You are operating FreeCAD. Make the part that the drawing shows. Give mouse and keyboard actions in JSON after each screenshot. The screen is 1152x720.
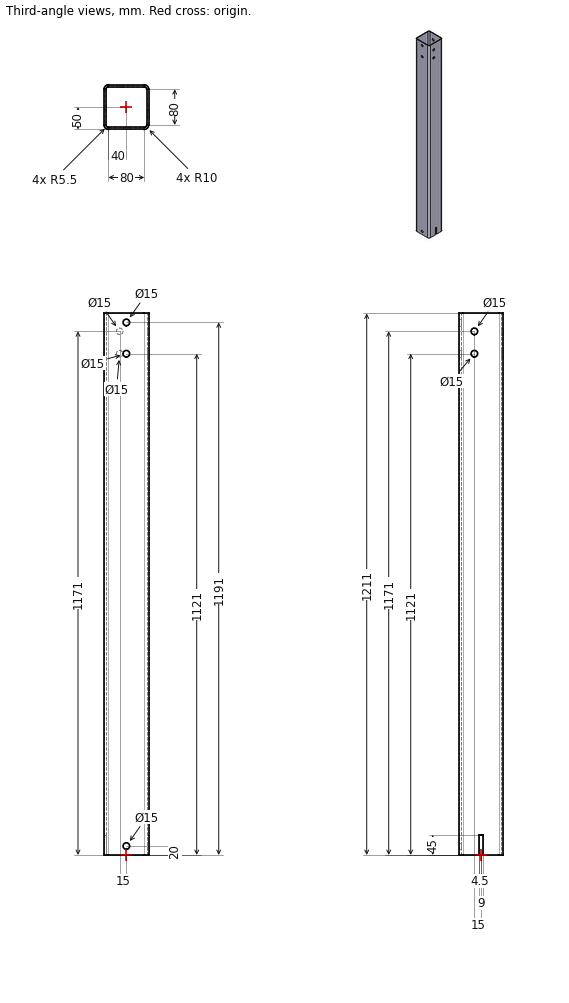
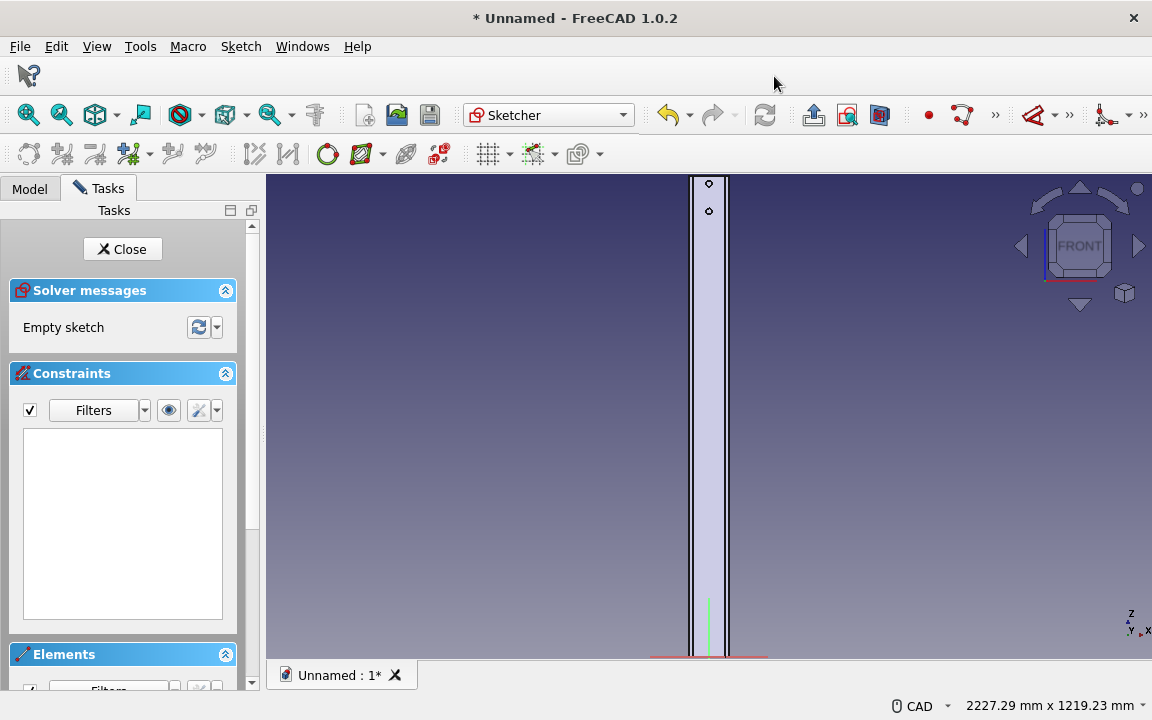
{"action": "scroll", "coordinate": [640, 416], "scroll_direction": "down", "scroll_amount": 5}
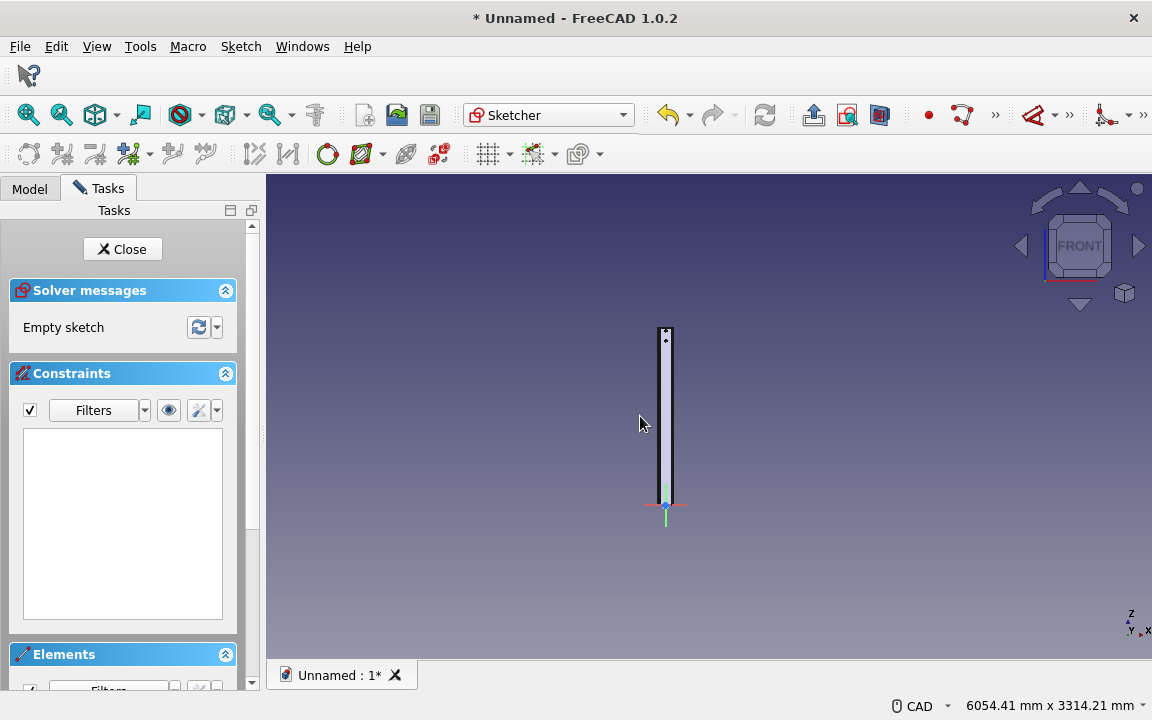
{"action": "scroll", "coordinate": [667, 508], "scroll_direction": "up", "scroll_amount": 15}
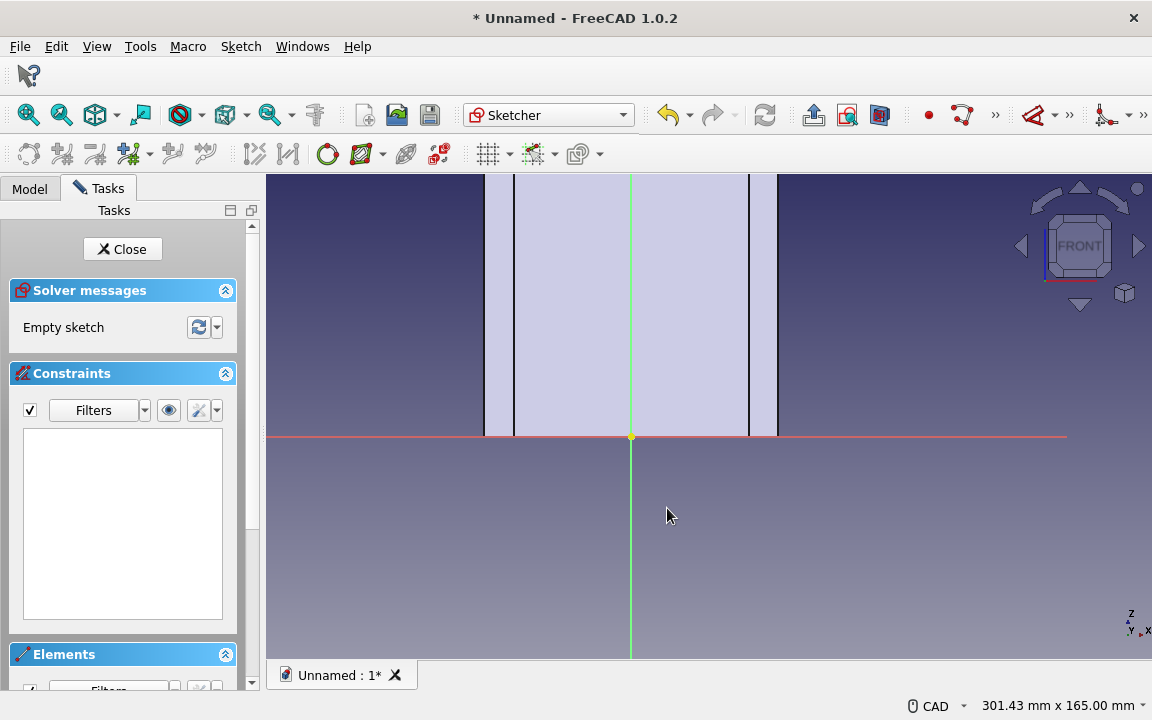
{"action": "scroll", "coordinate": [628, 390], "scroll_direction": "up", "scroll_amount": 7}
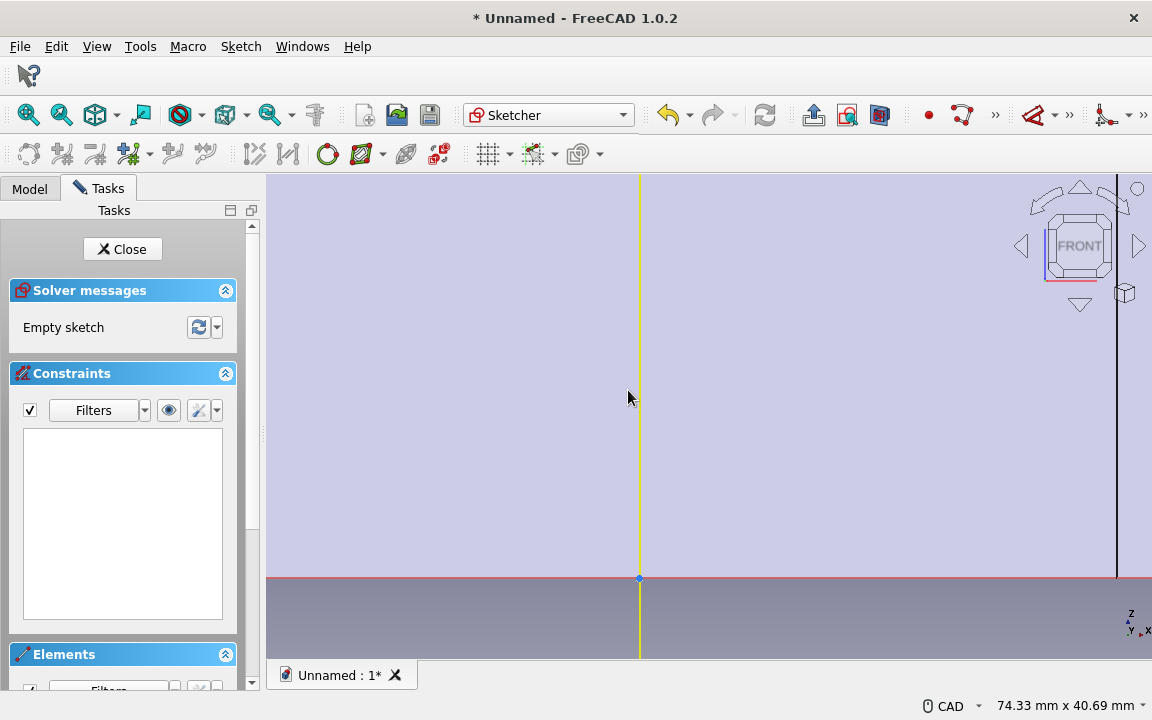
{"action": "key", "text": "g c"}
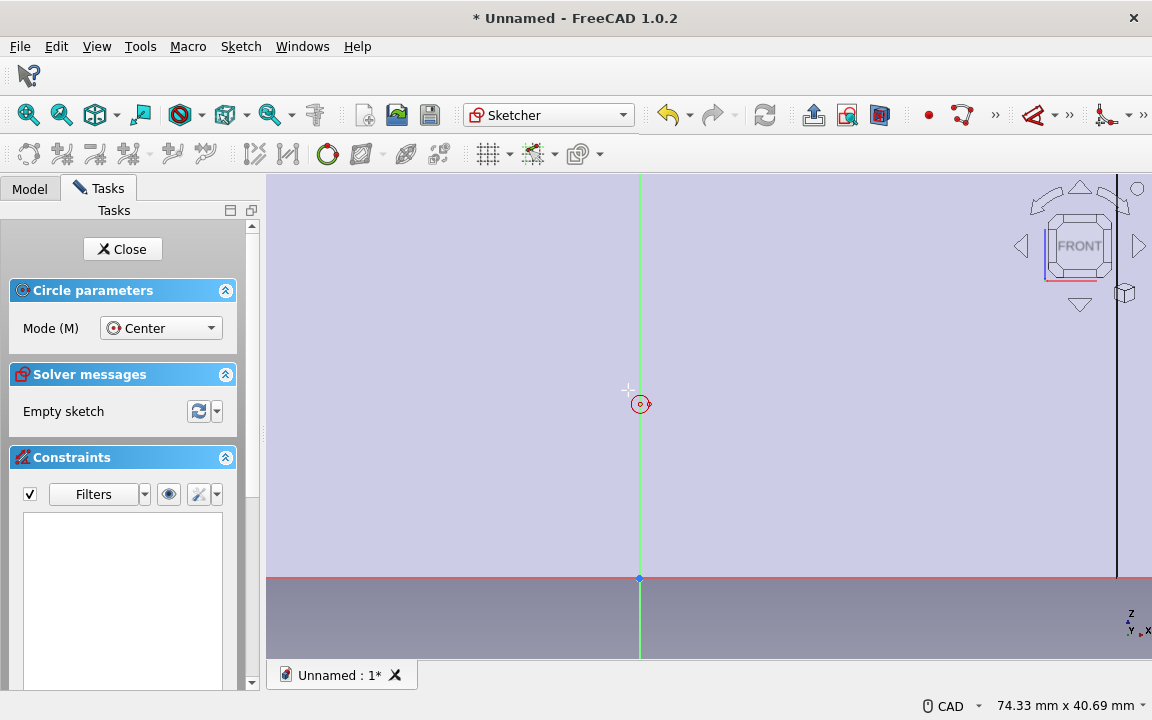
{"action": "left_click", "coordinate": [640, 340]}
{"action": "left_click", "coordinate": [703, 277]}
{"action": "key", "text": "Escape"}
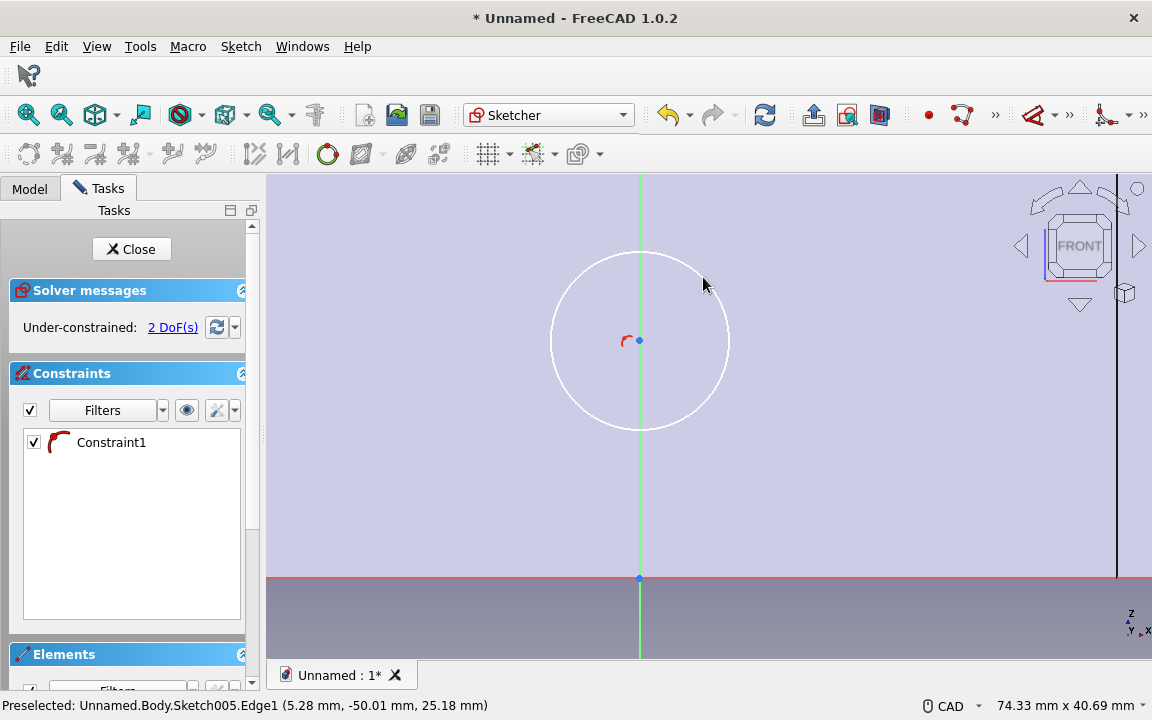
{"action": "key", "text": "d"}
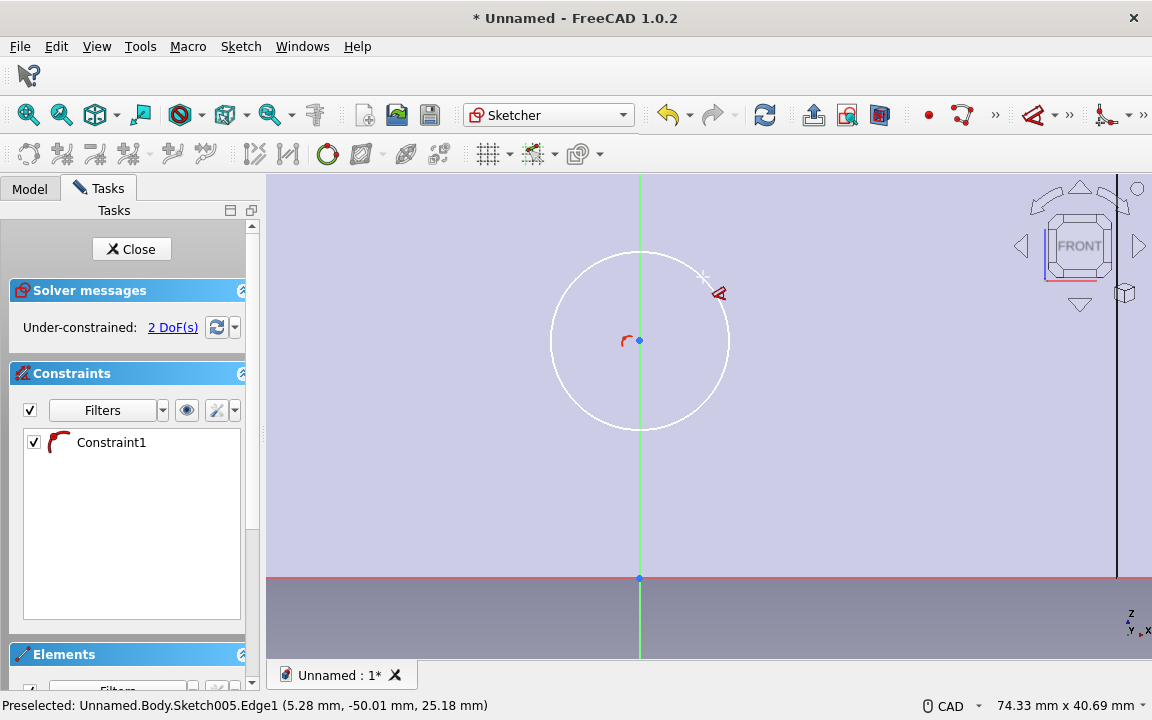
{"action": "left_click", "coordinate": [703, 278]}
{"action": "left_click", "coordinate": [726, 255]}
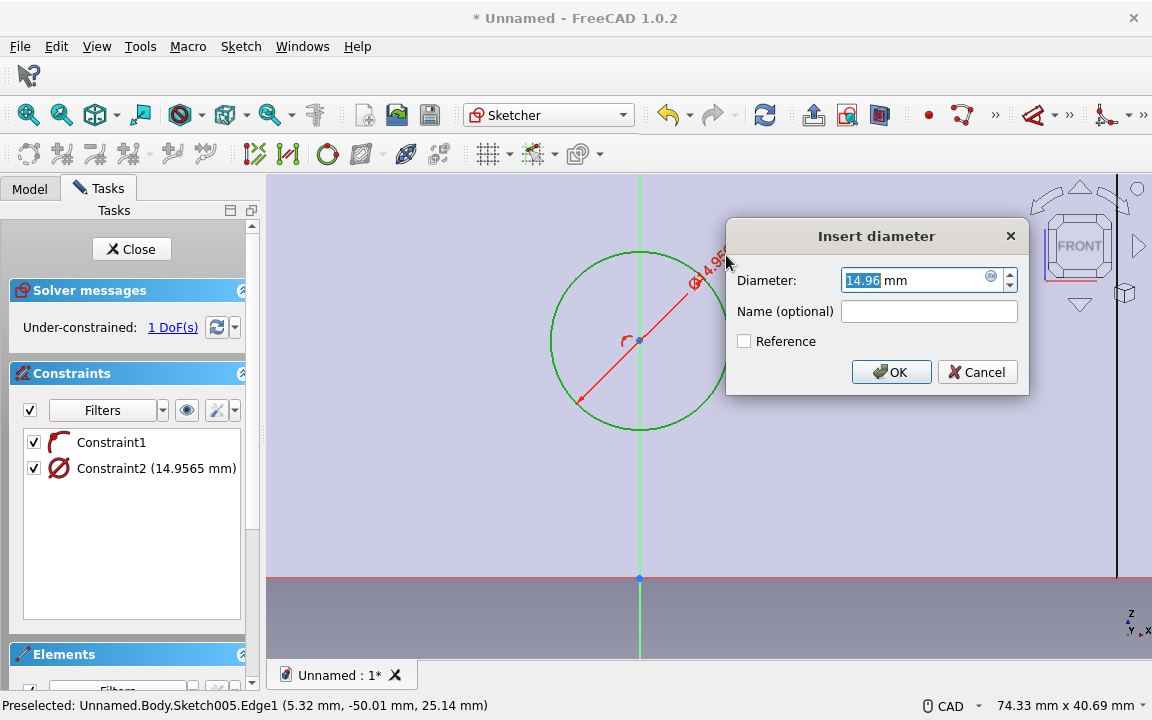
{"action": "type", "text": "15"}
{"action": "key", "text": "Return"}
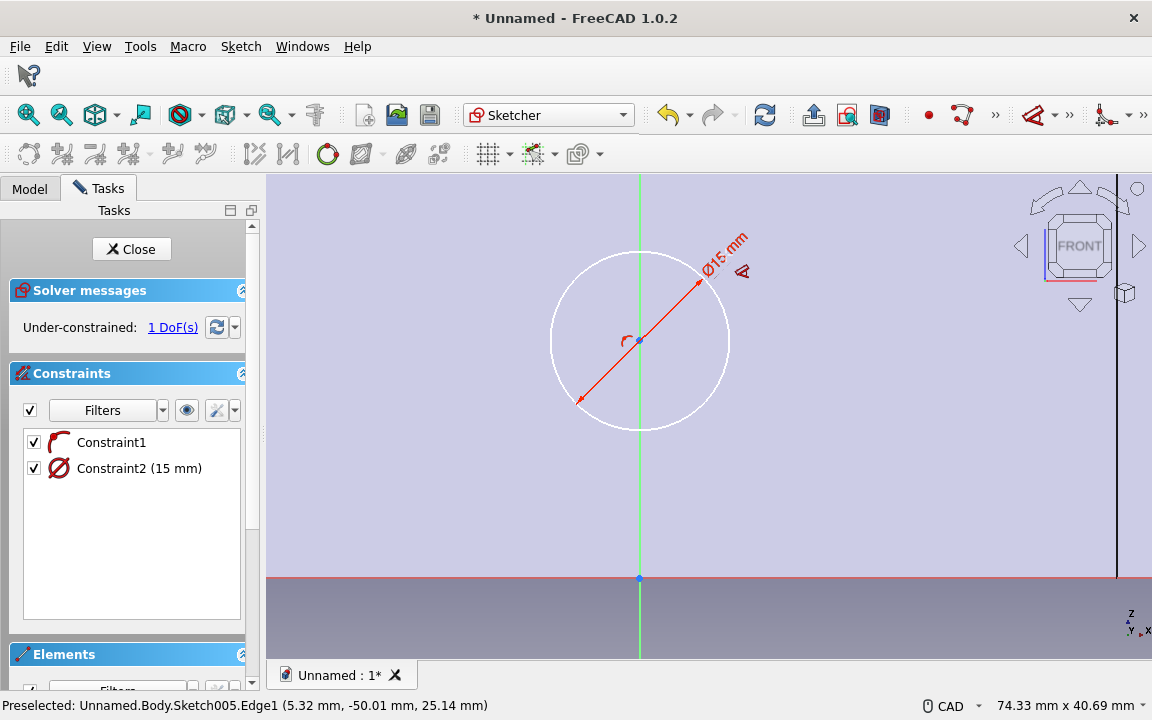
{"action": "left_click", "coordinate": [640, 341]}
{"action": "left_click", "coordinate": [674, 460]}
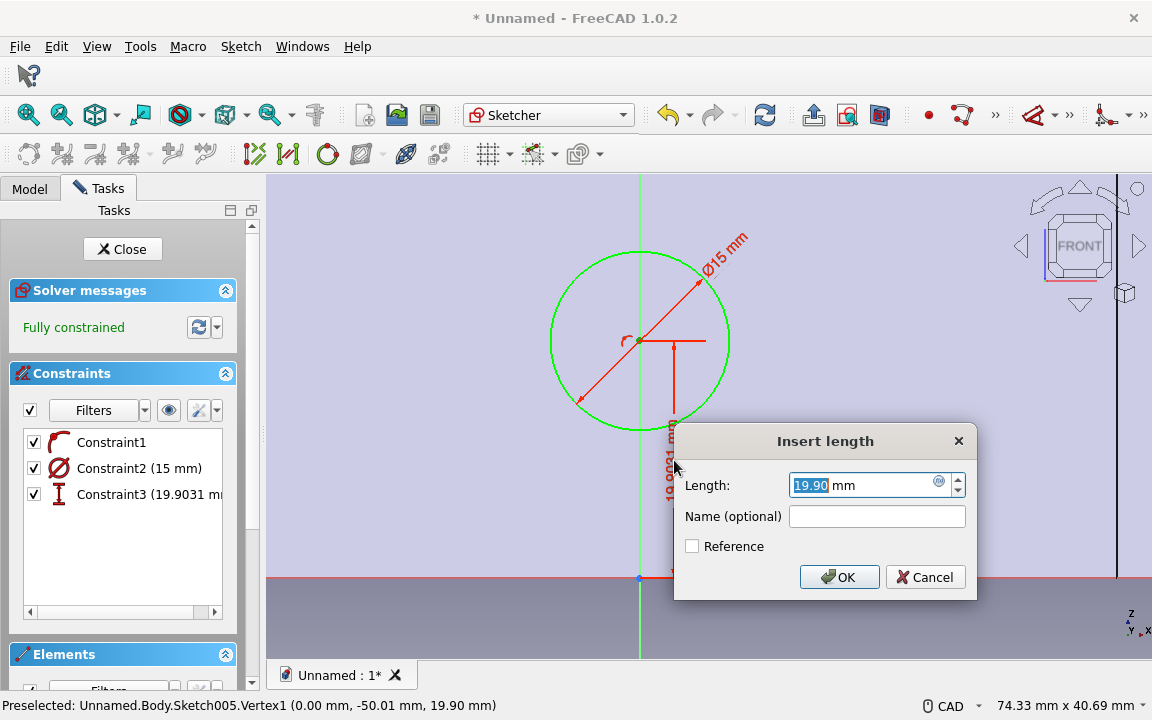
{"action": "type", "text": "20"}
{"action": "key", "text": "Return"}
{"action": "key", "text": "Escape"}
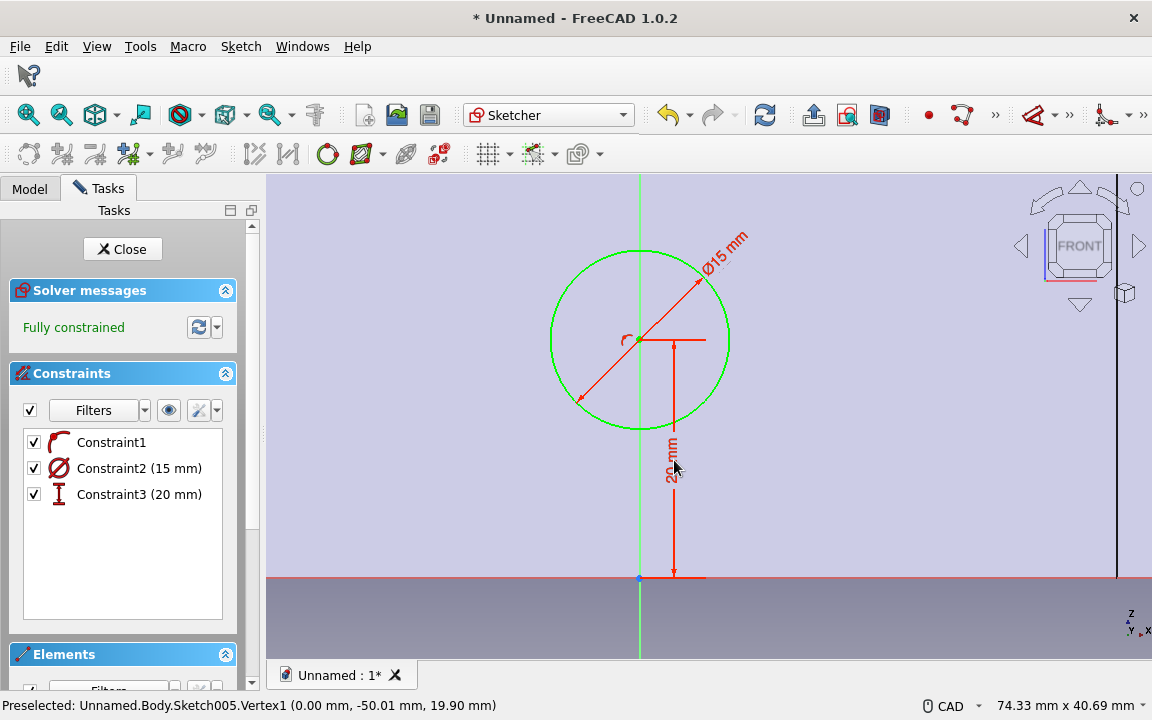
{"action": "left_click", "coordinate": [123, 249]}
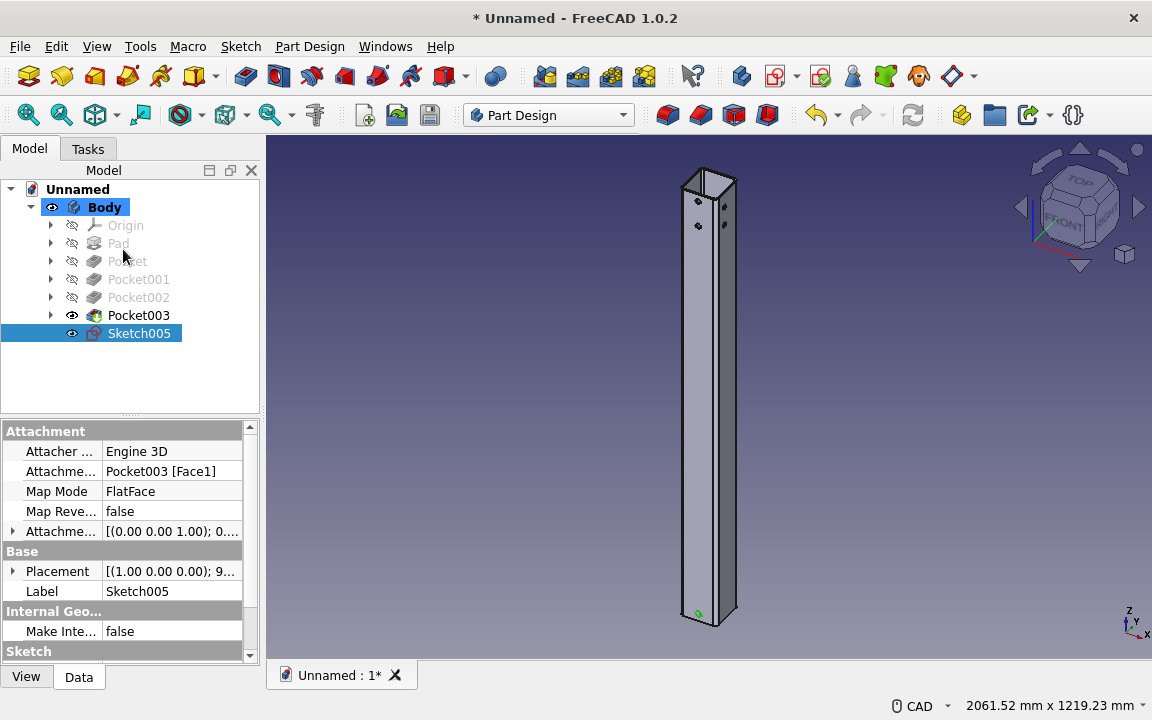
{"action": "left_click", "coordinate": [246, 76]}